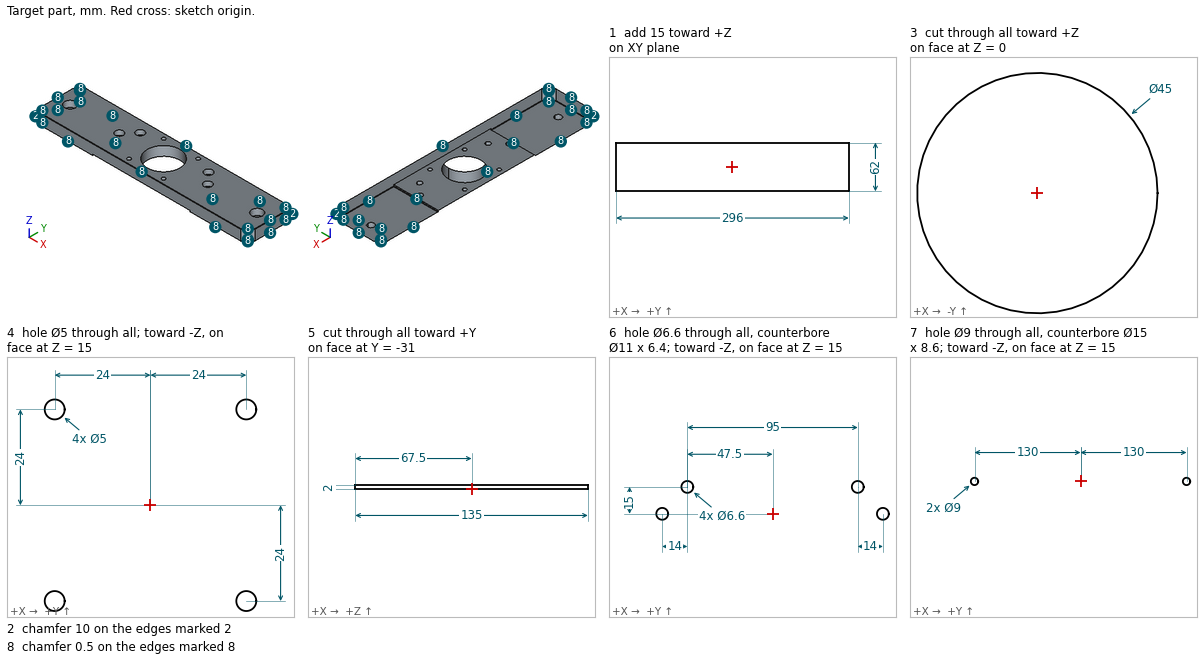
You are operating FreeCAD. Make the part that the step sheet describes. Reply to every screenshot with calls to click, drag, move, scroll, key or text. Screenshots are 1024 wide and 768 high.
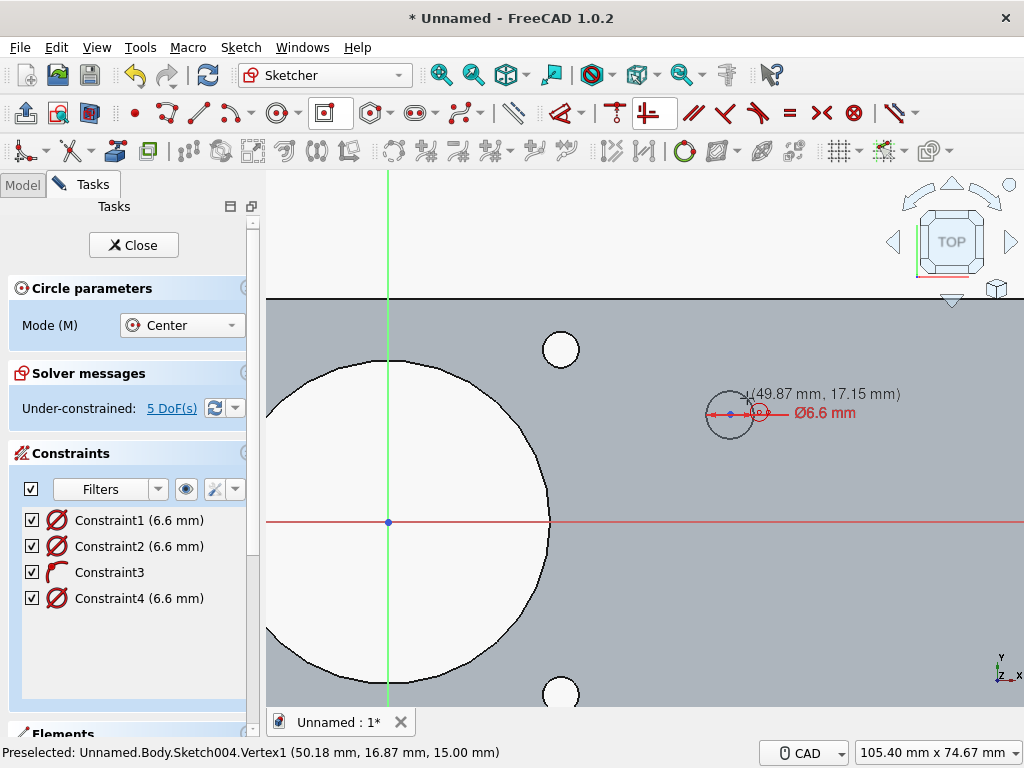
click(831, 522)
move(847, 506)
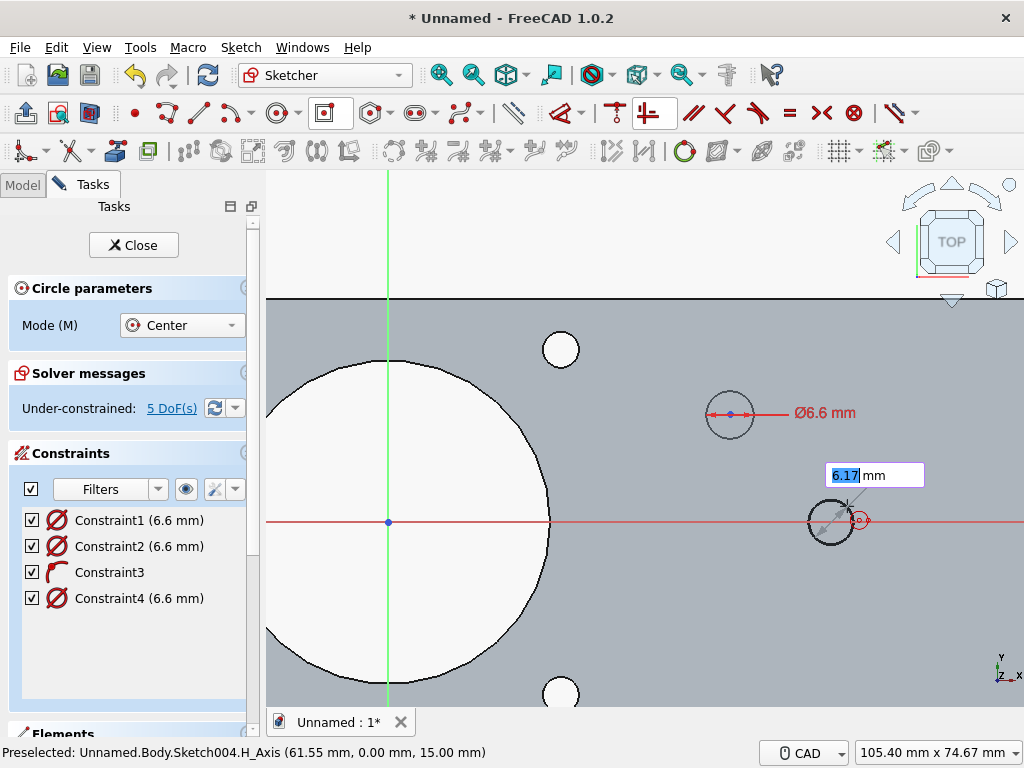
text(6.6)
key(Return)
key(Escape)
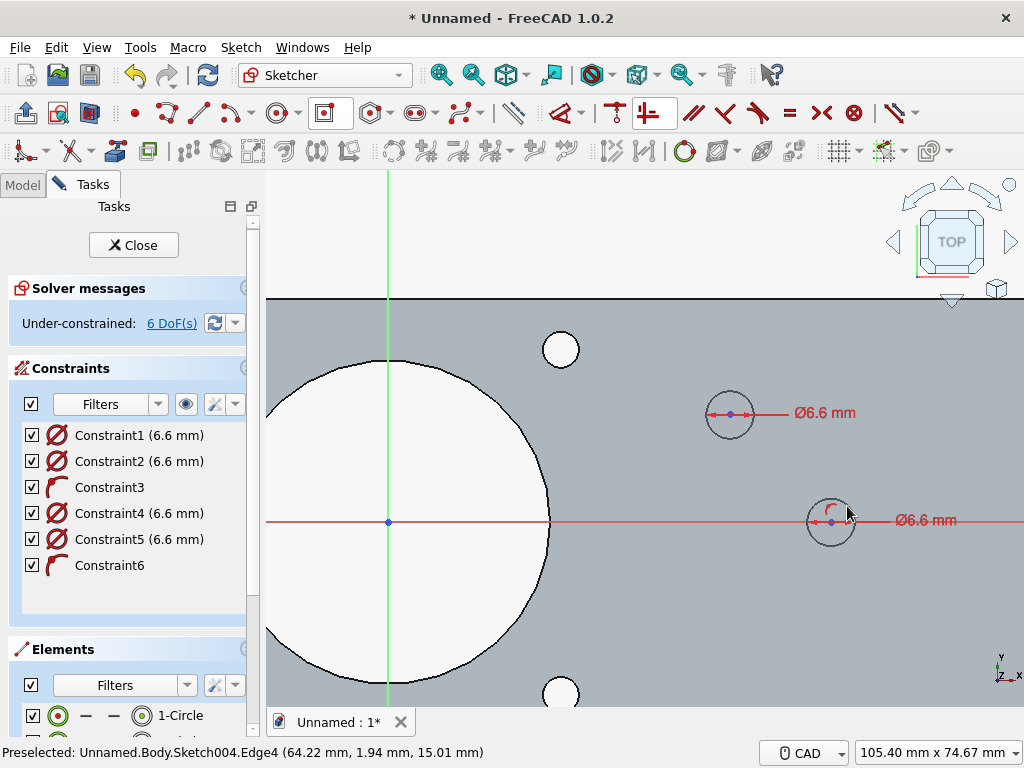
scroll(730, 414, down, 4)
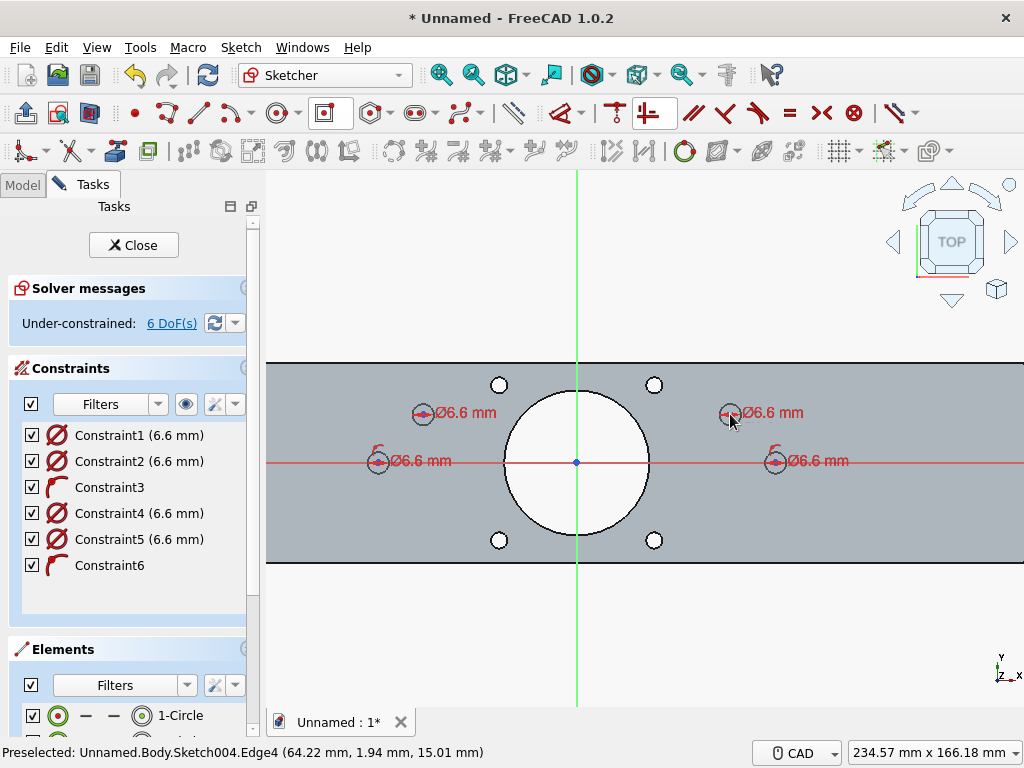
click(423, 415)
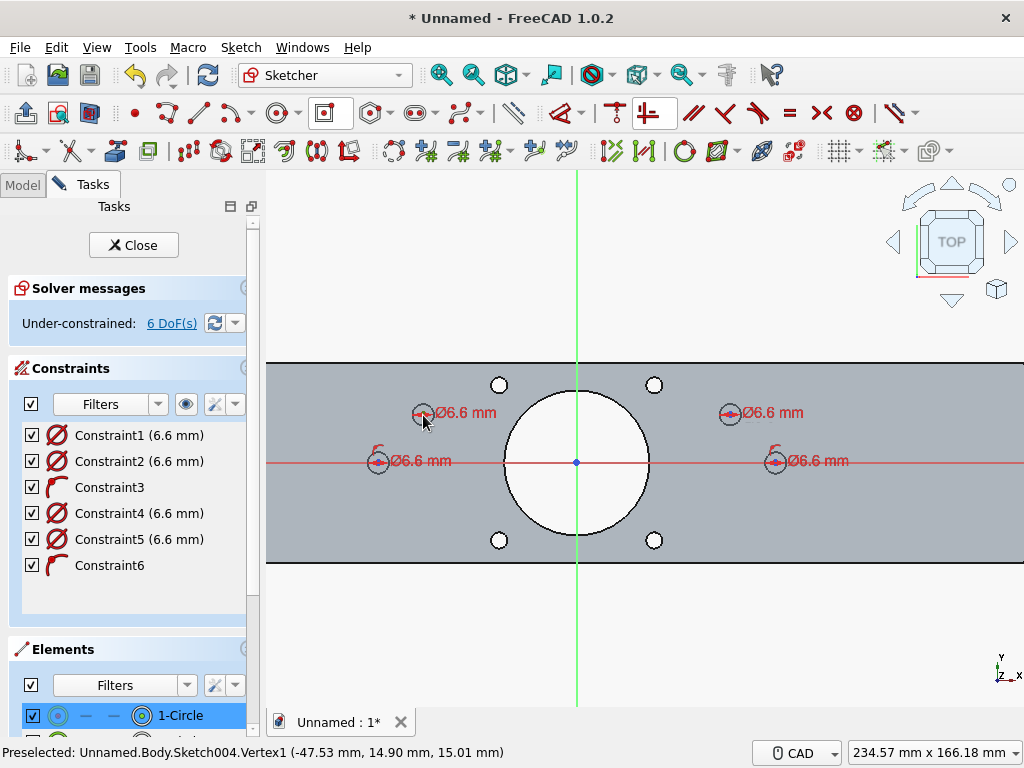
click(730, 415)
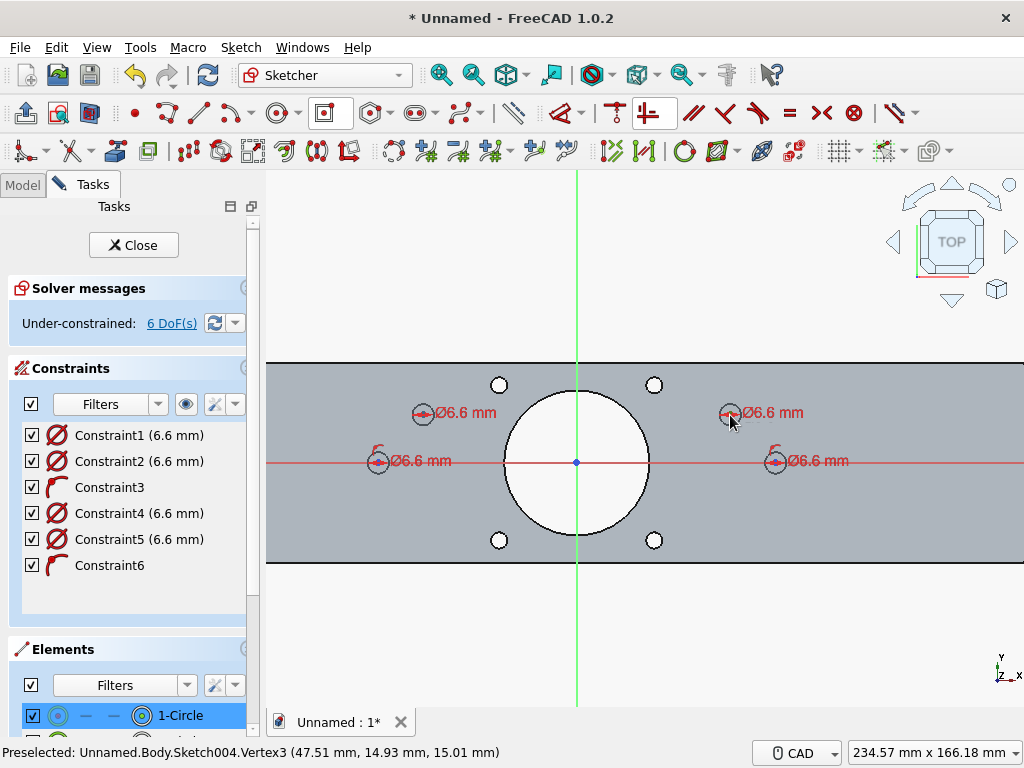
click(672, 114)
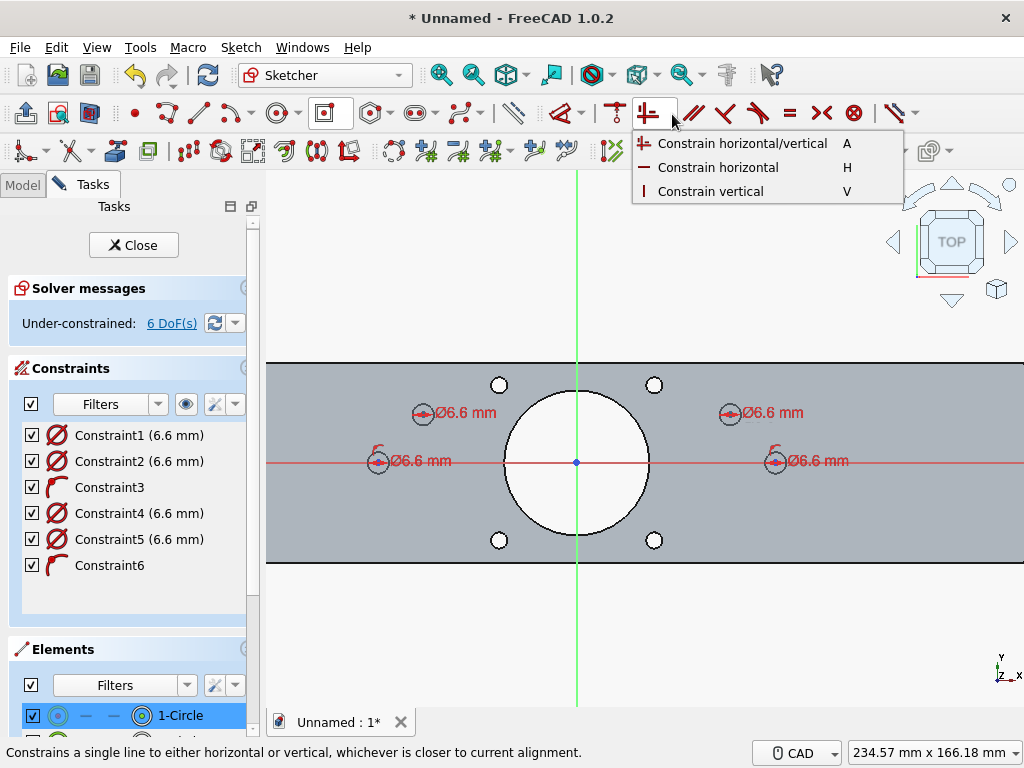
click(768, 167)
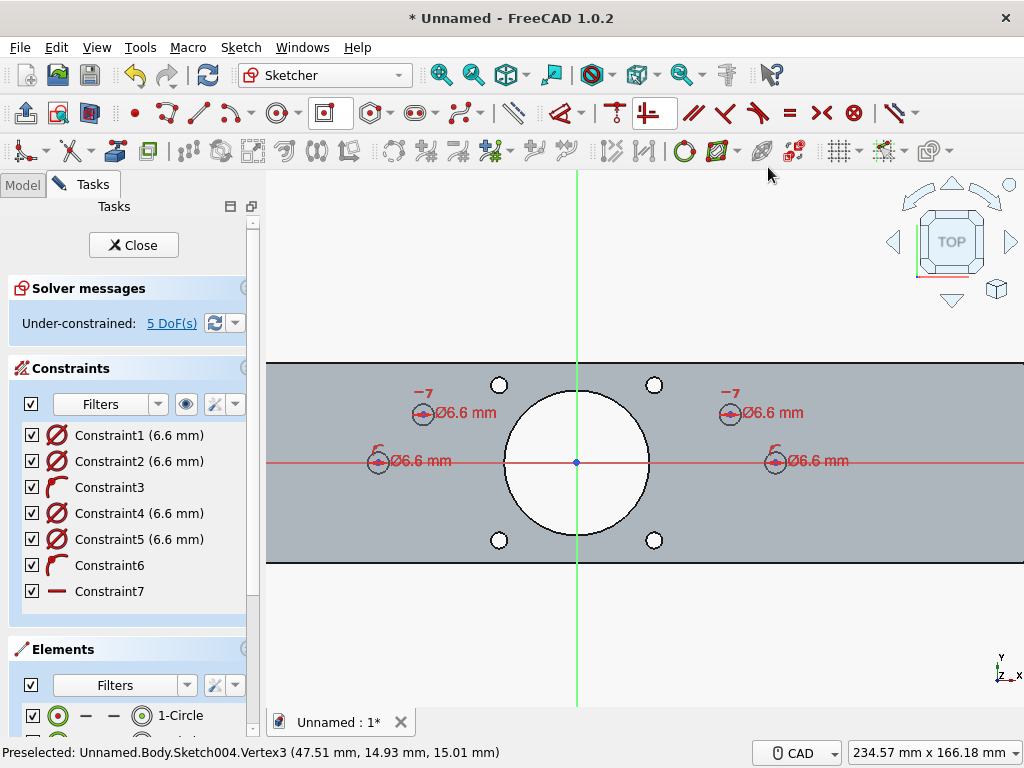
click(560, 114)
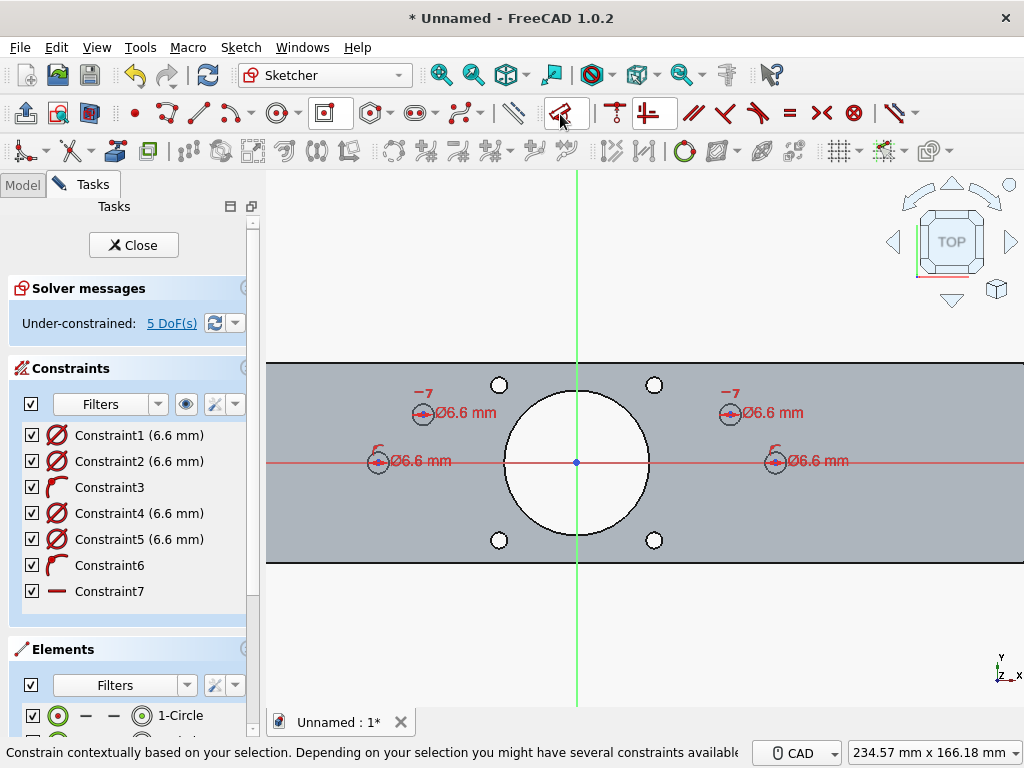
click(423, 415)
click(389, 439)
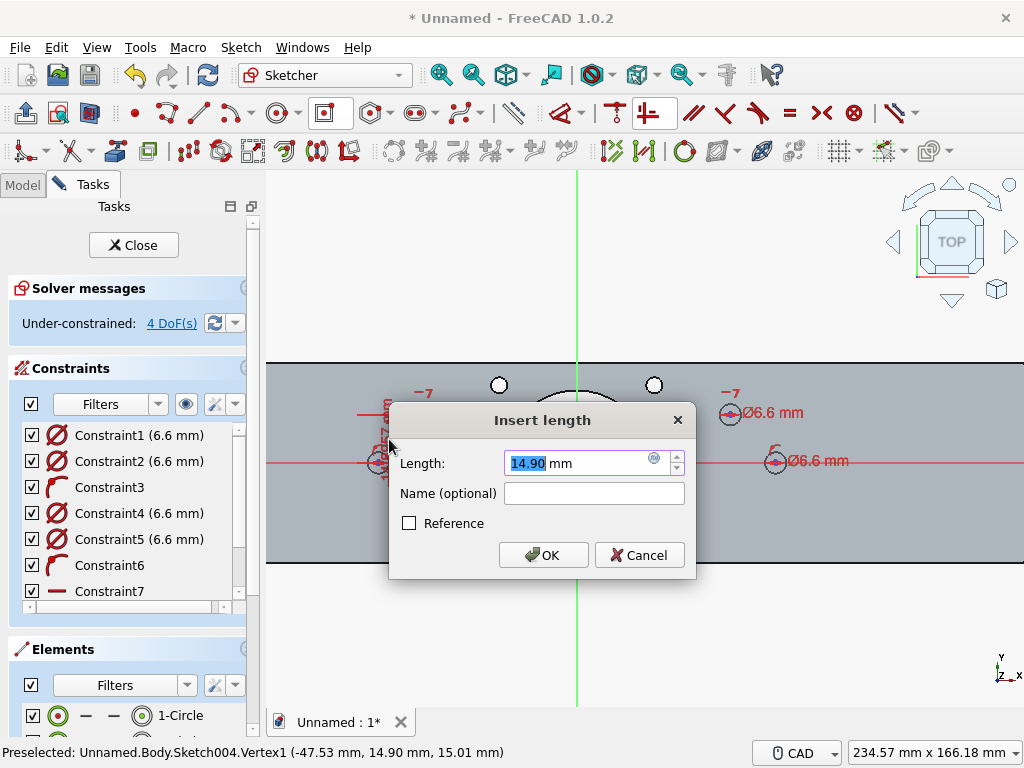
text(15)
key(Return)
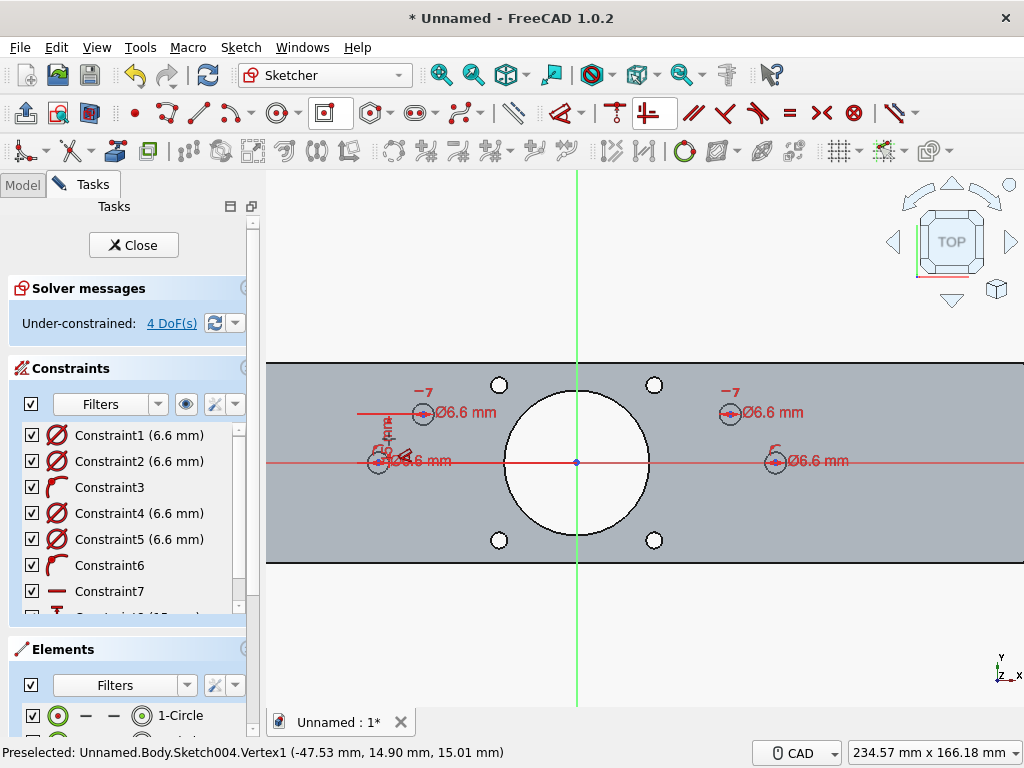
click(423, 414)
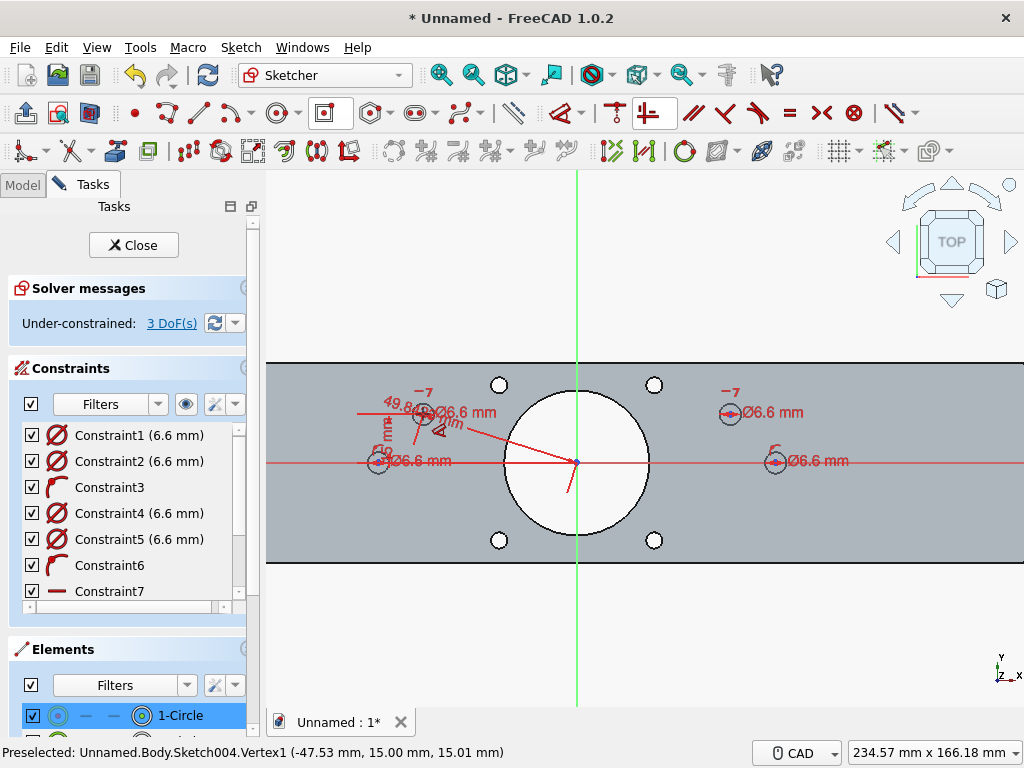
click(378, 463)
click(401, 497)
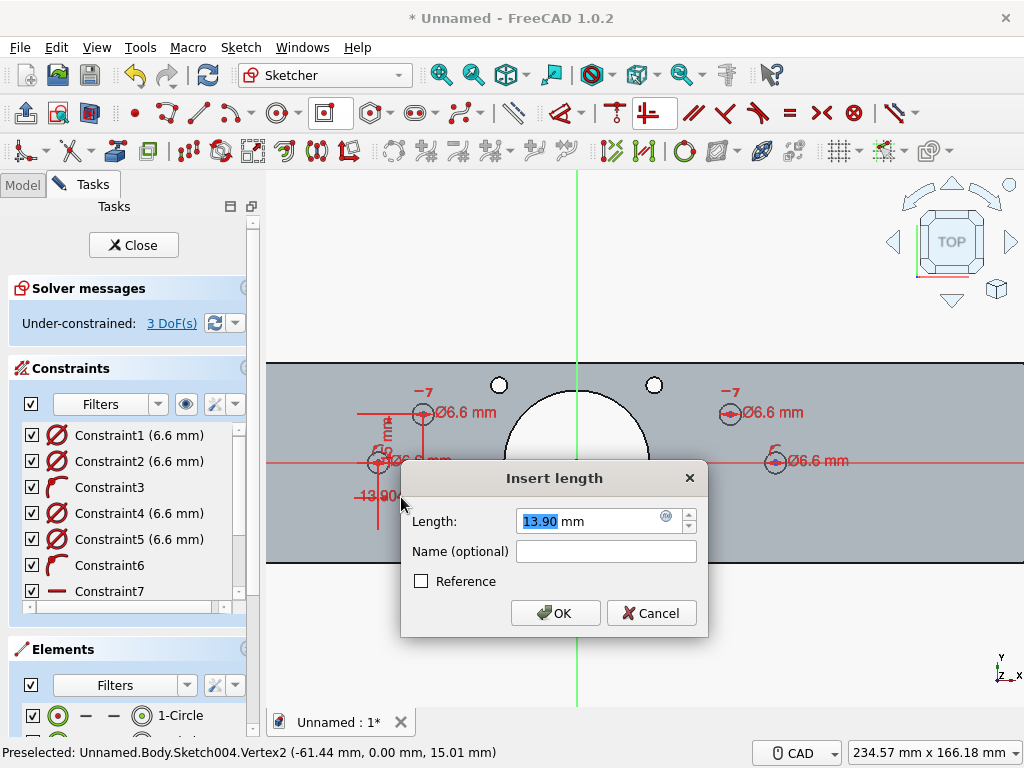
text(14)
key(Return)